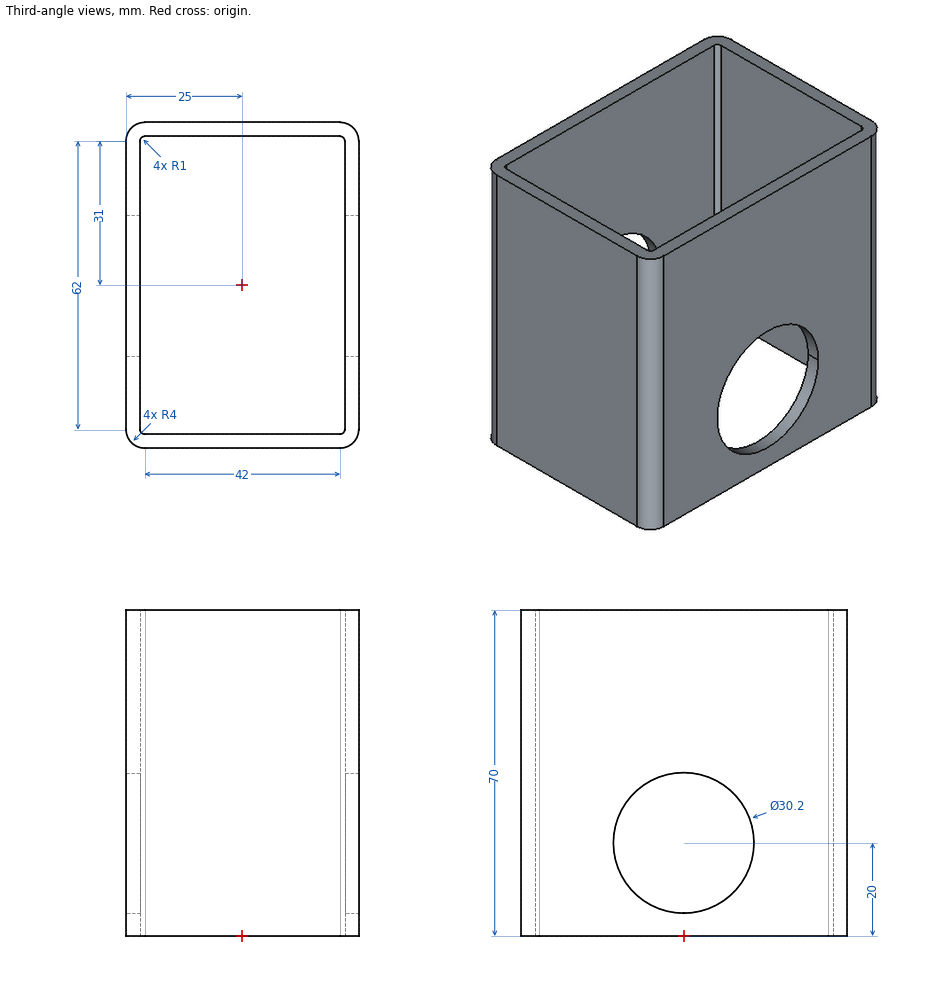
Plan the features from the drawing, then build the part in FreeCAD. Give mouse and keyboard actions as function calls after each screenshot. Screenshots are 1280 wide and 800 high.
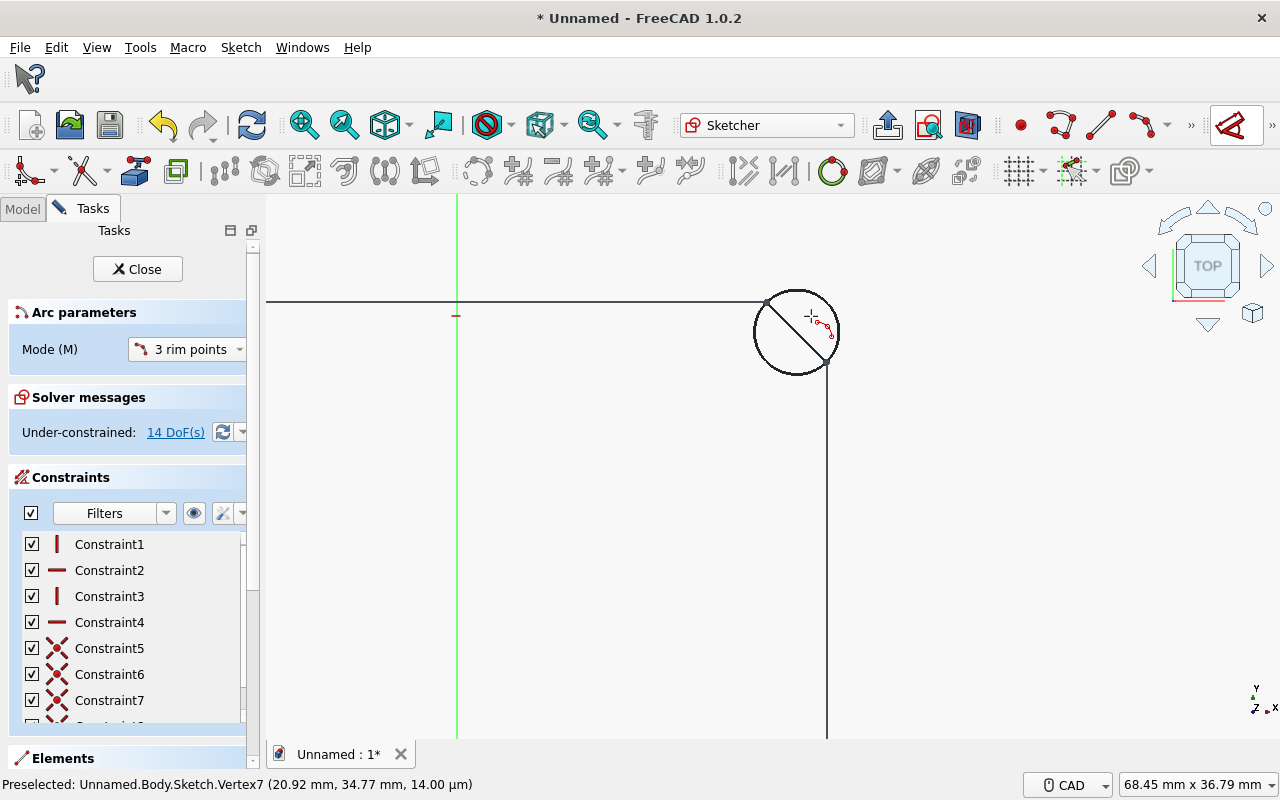
click(810, 316)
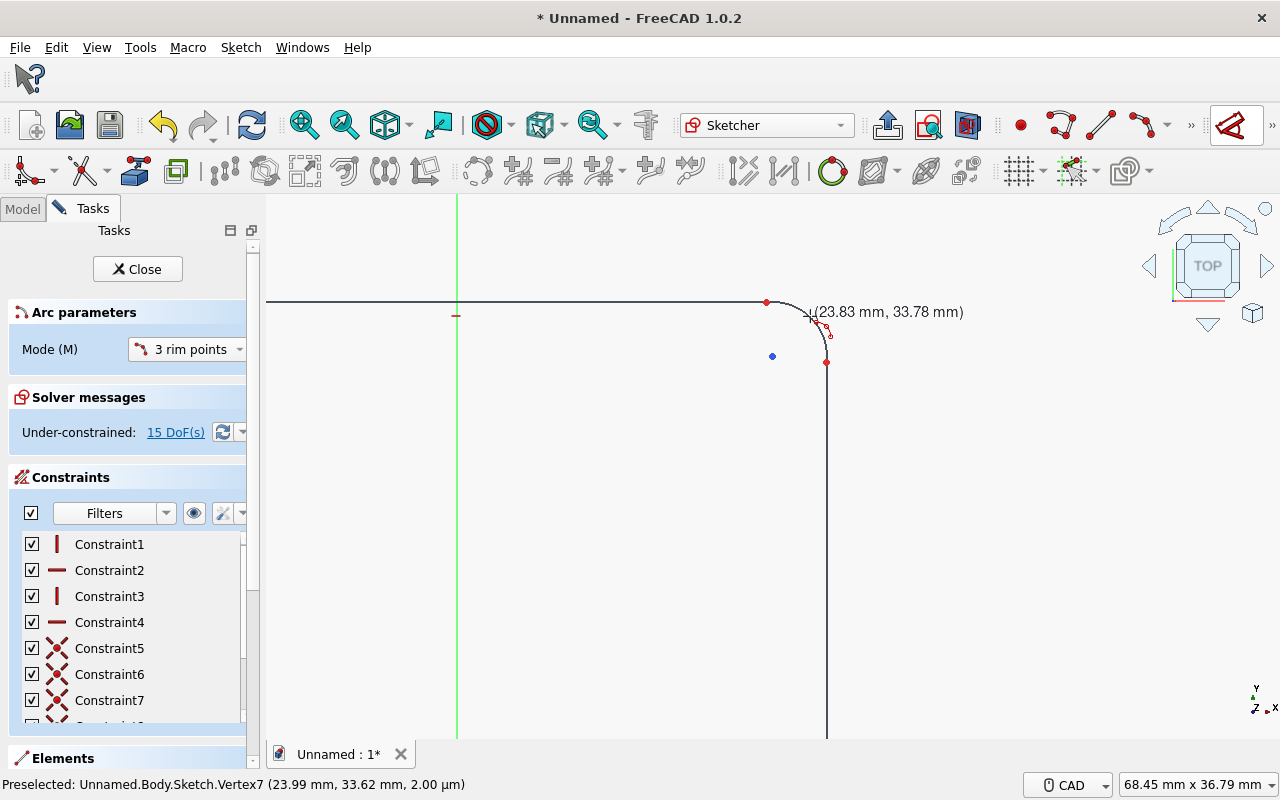
scroll(811, 315, down, 6)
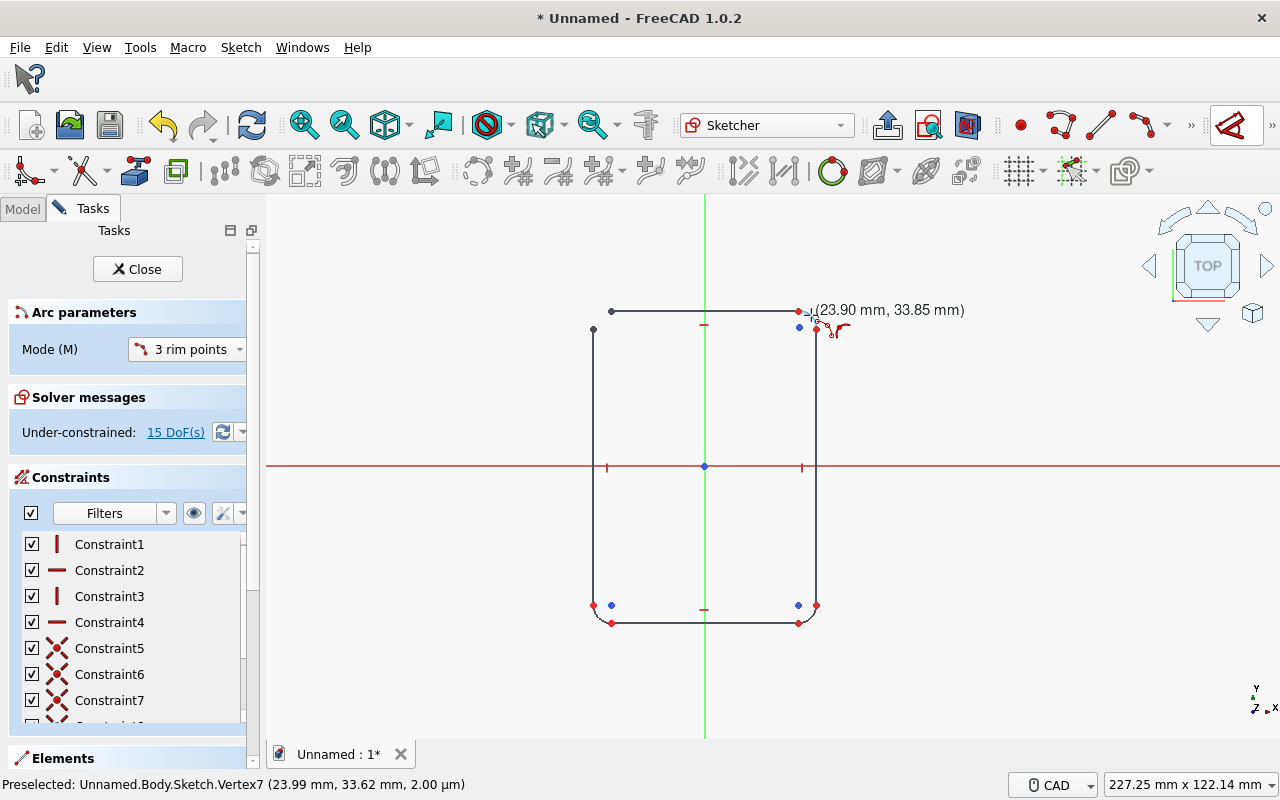
click(611, 311)
click(593, 329)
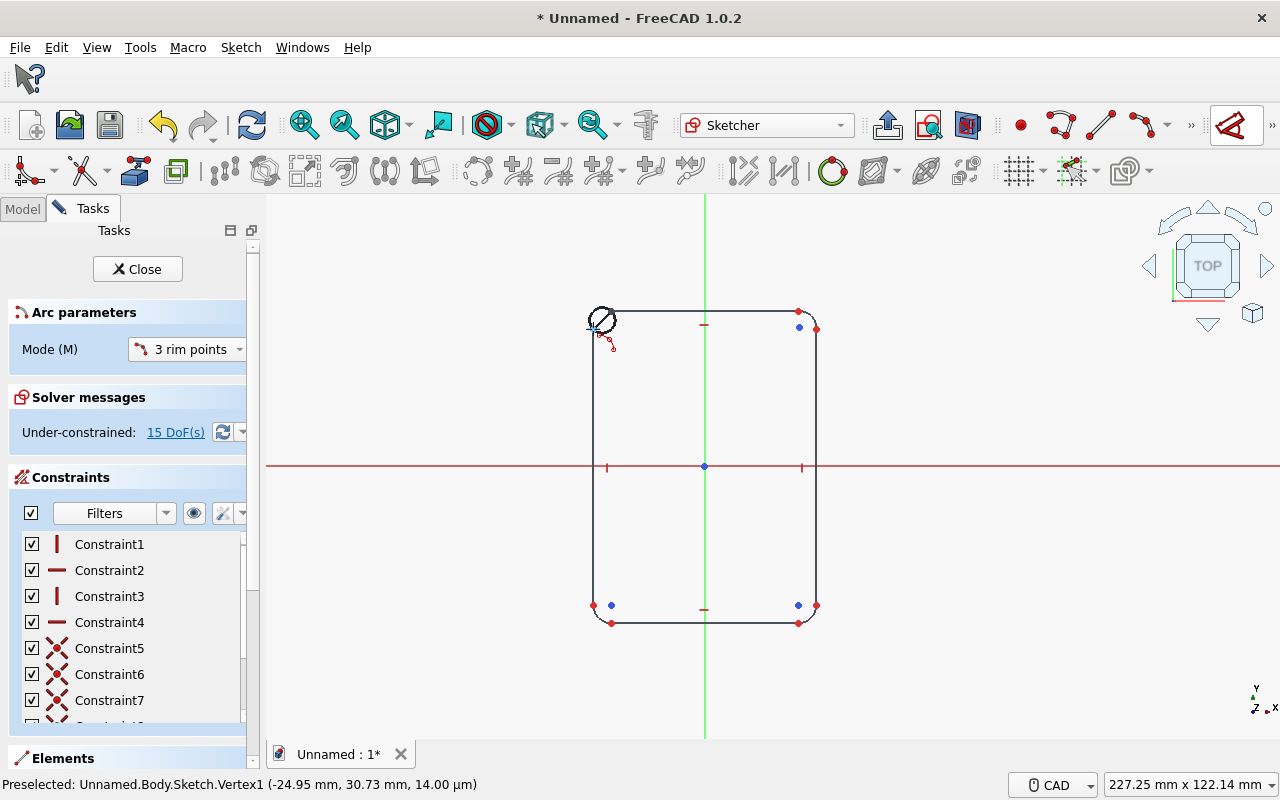
scroll(598, 316, up, 6)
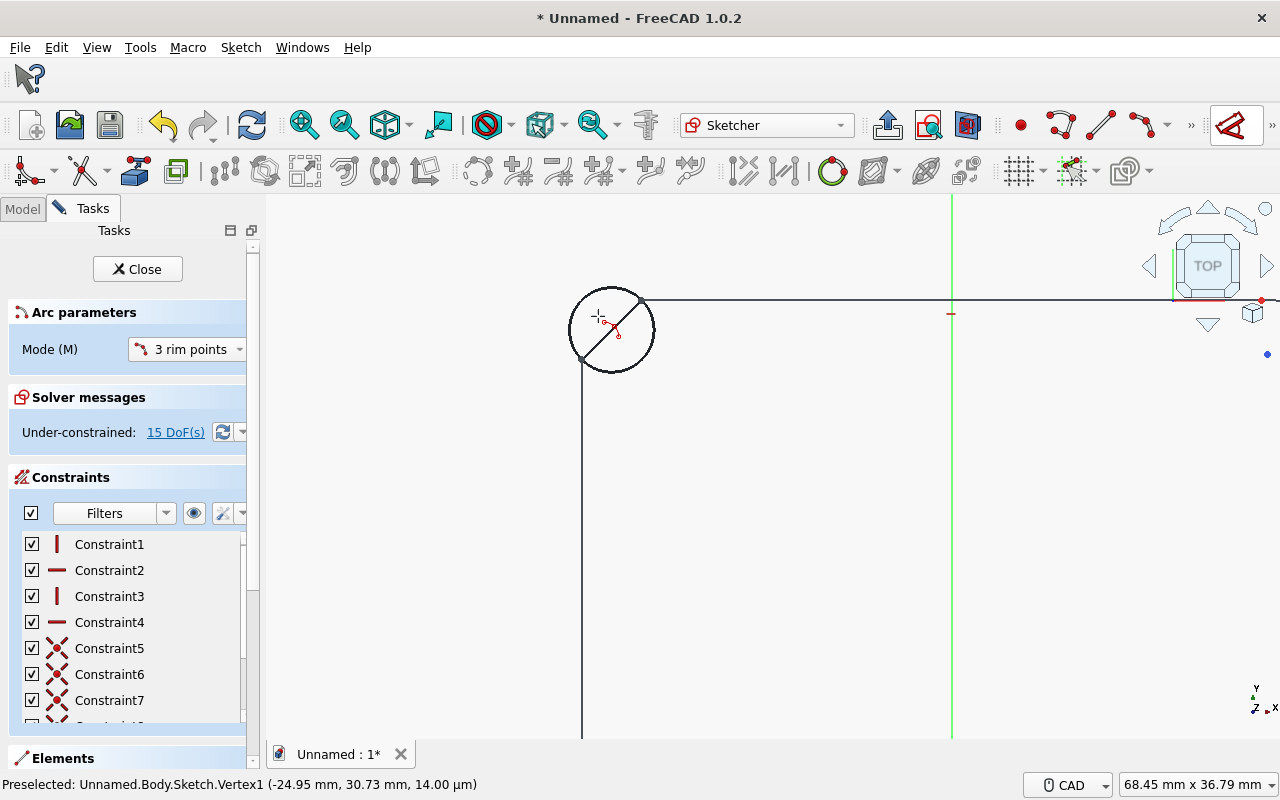
click(599, 314)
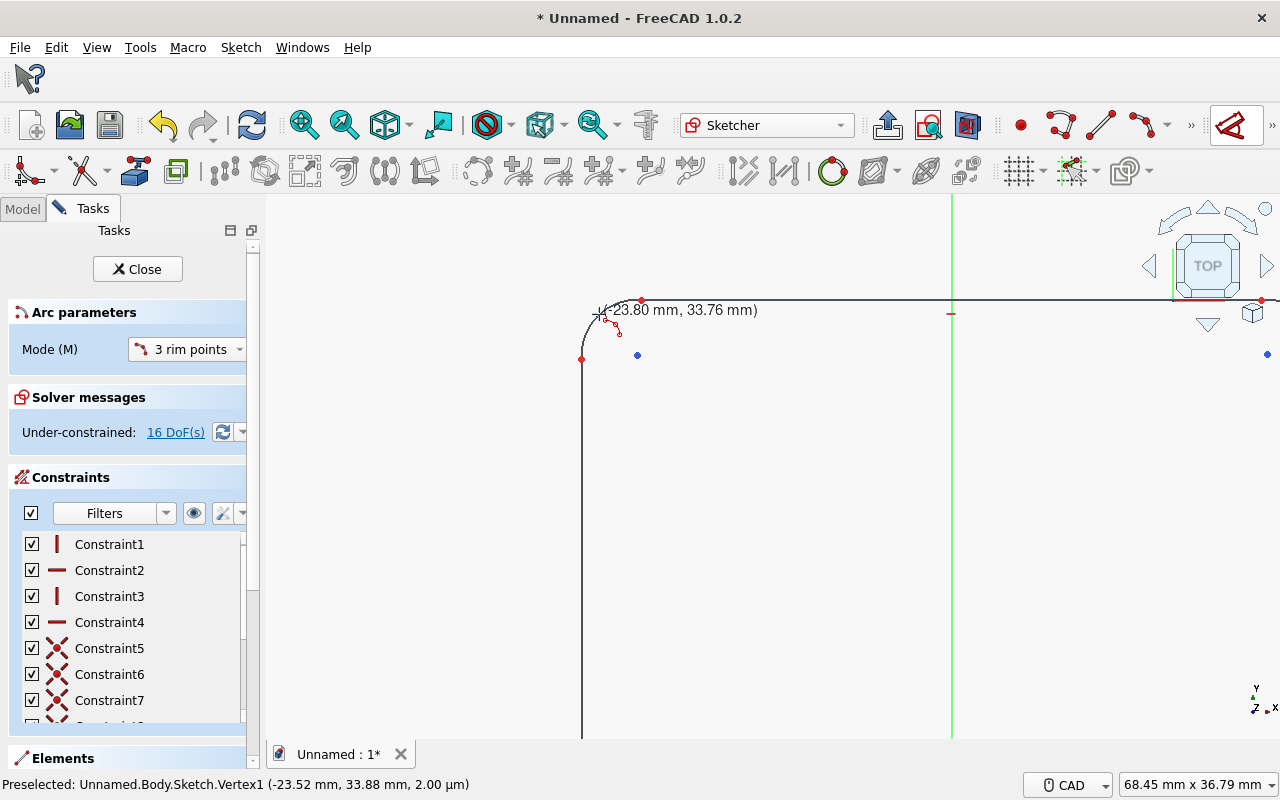
key(g)
key(l)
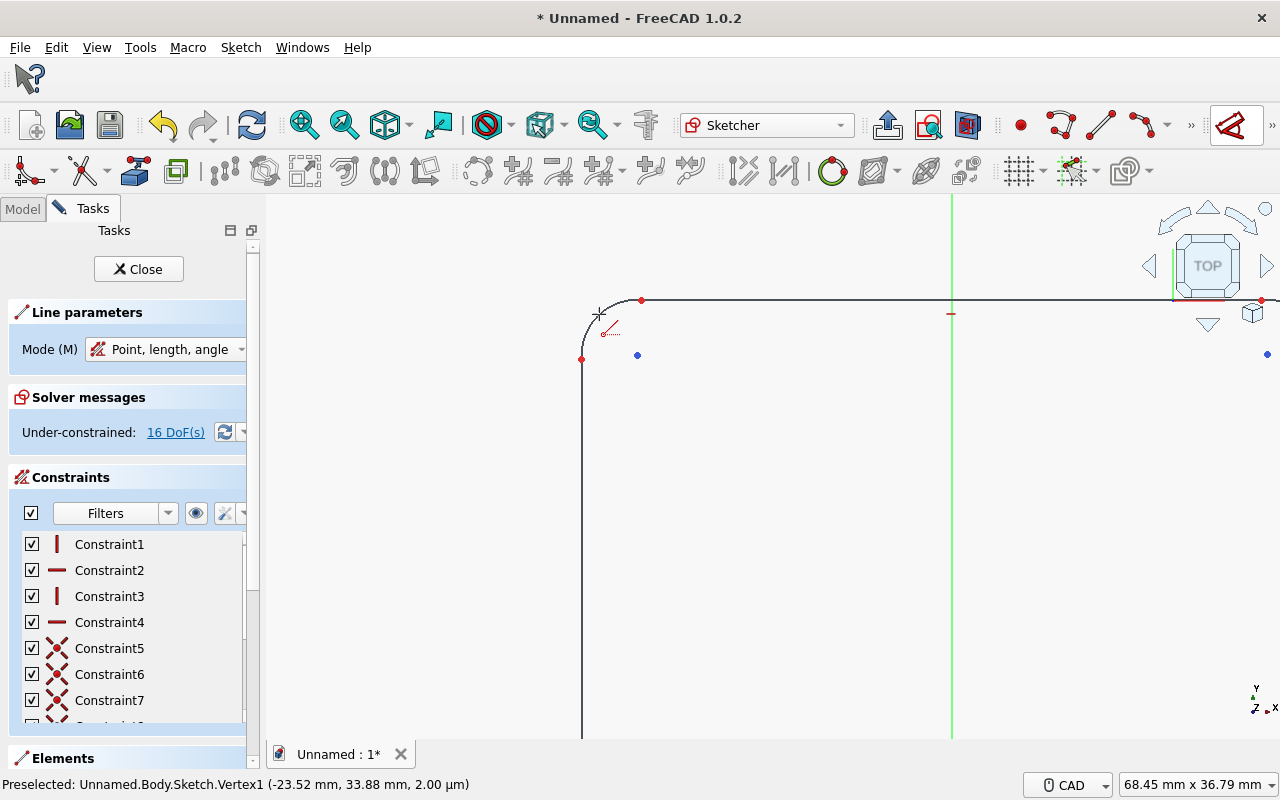
scroll(598, 316, down, 6)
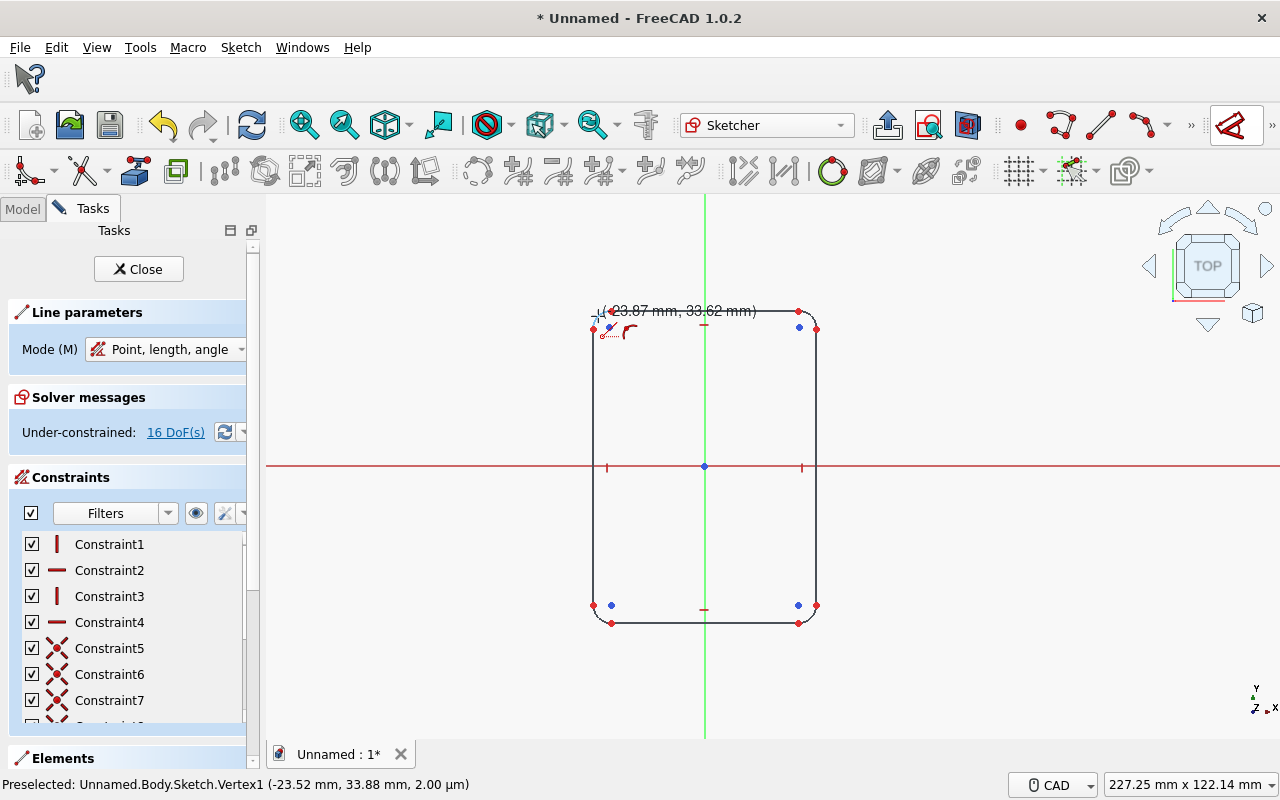
scroll(607, 605, up, 7)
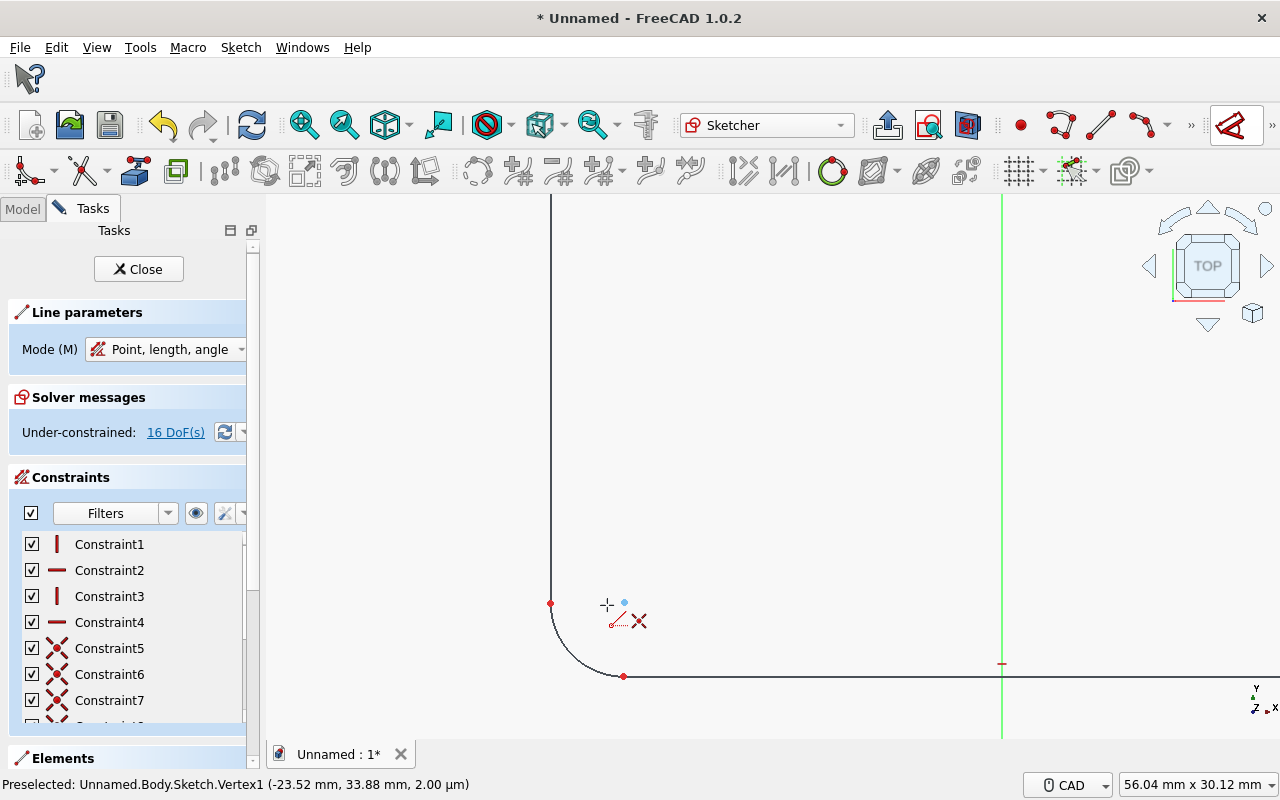
click(604, 602)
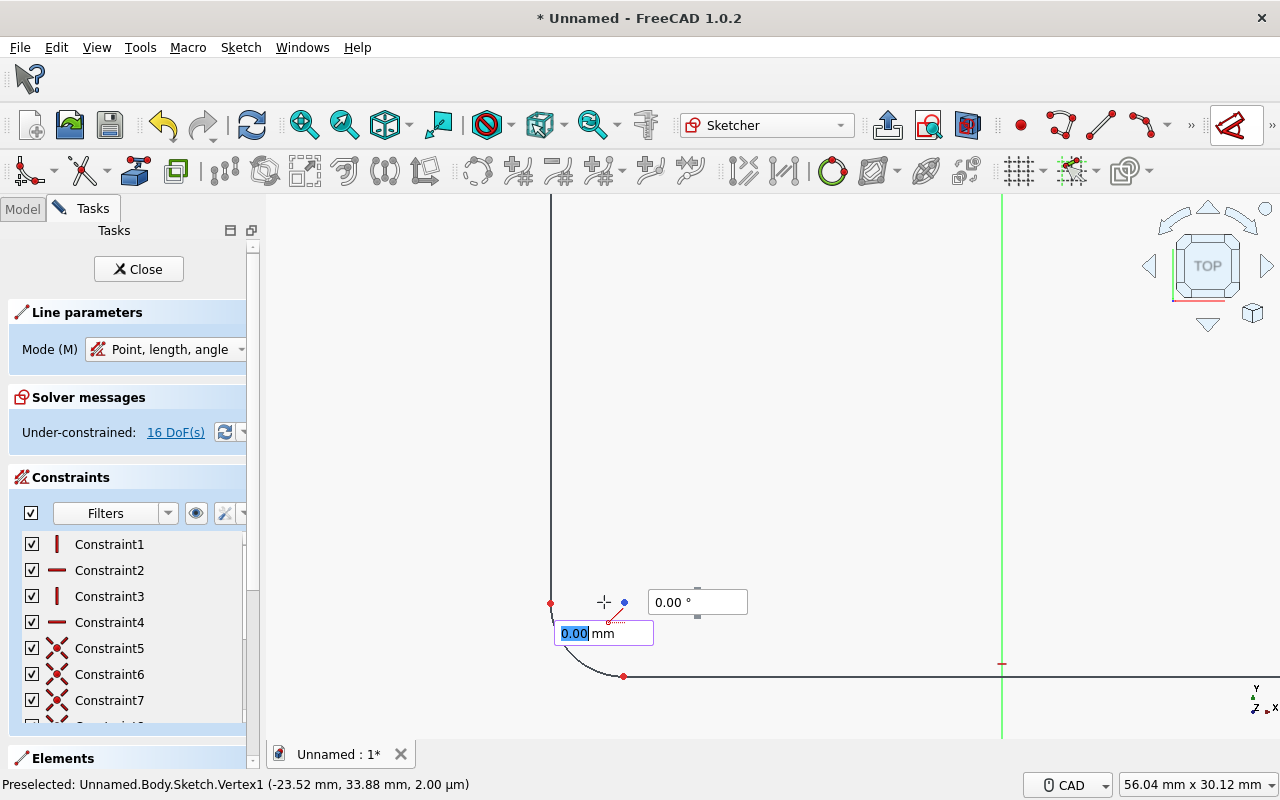
scroll(607, 606, down, 7)